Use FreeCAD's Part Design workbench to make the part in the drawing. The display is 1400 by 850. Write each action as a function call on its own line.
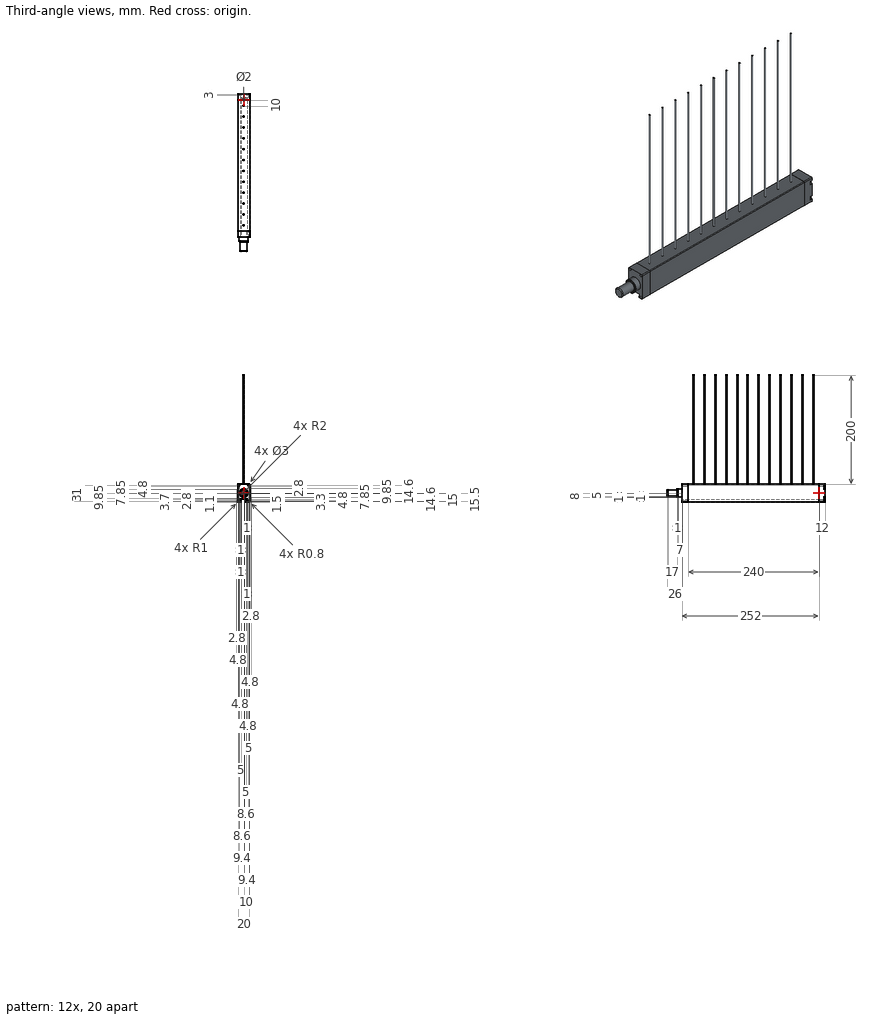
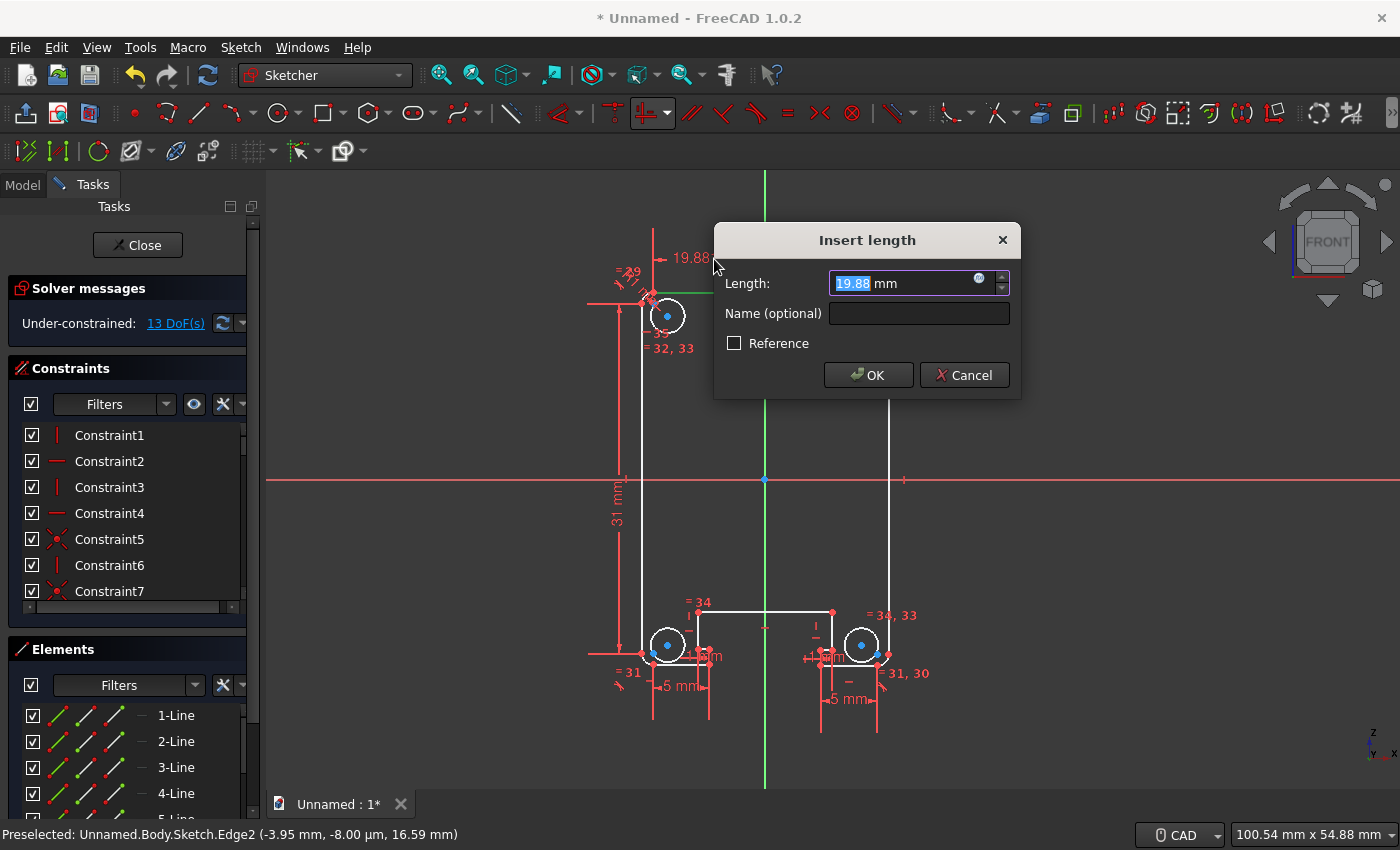
text(20)
key(Return)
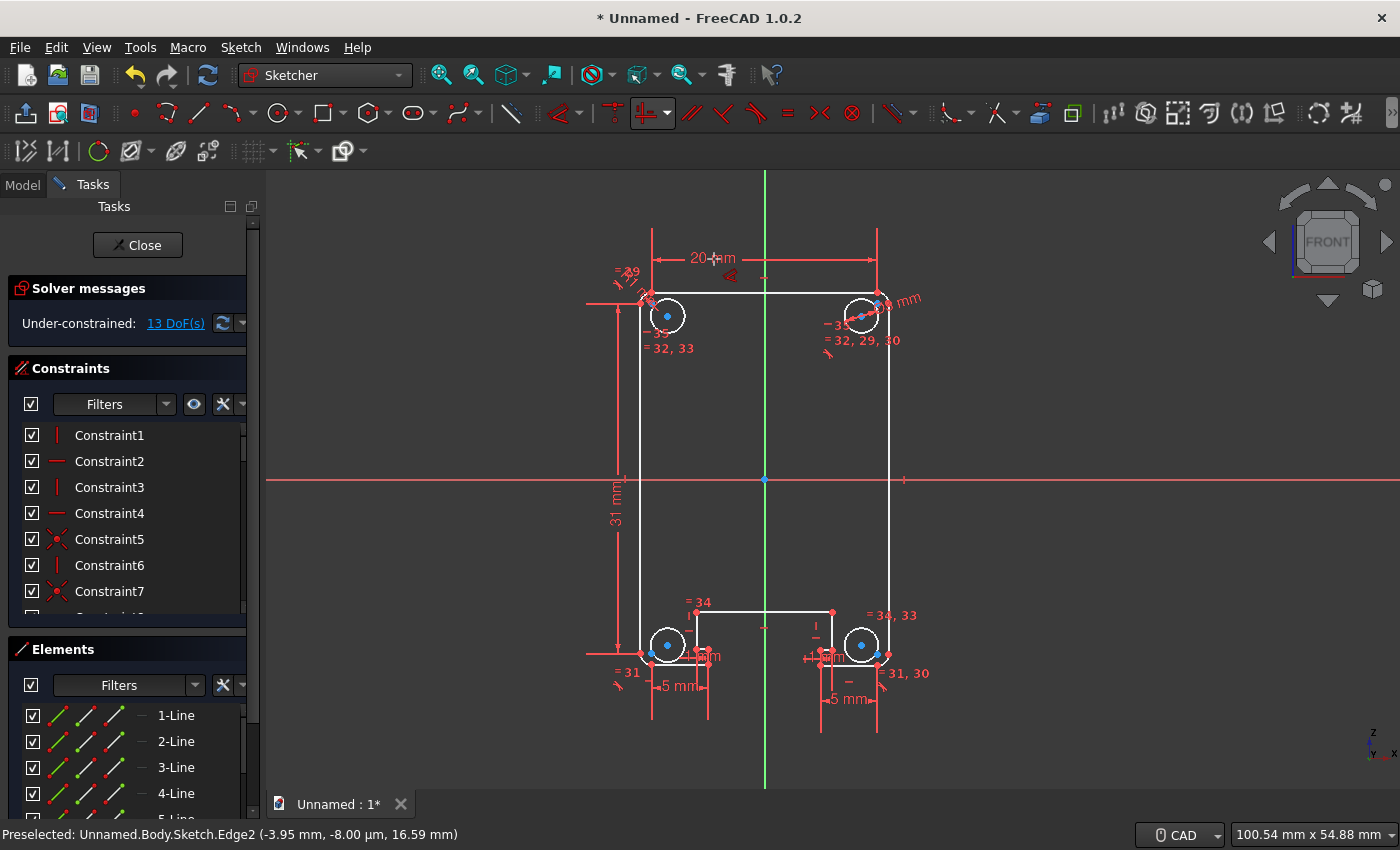
click(889, 409)
click(923, 399)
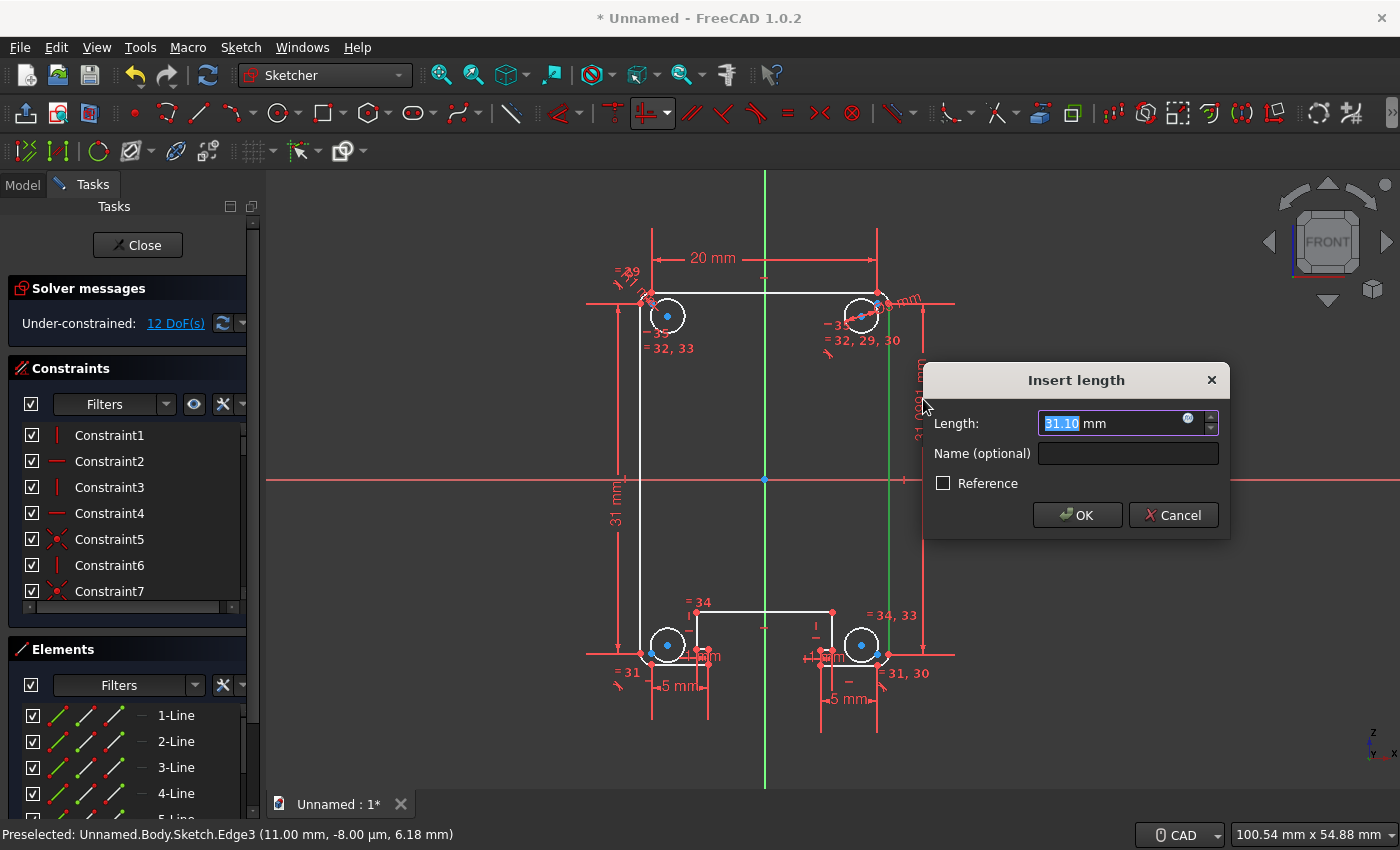
text(31)
key(Return)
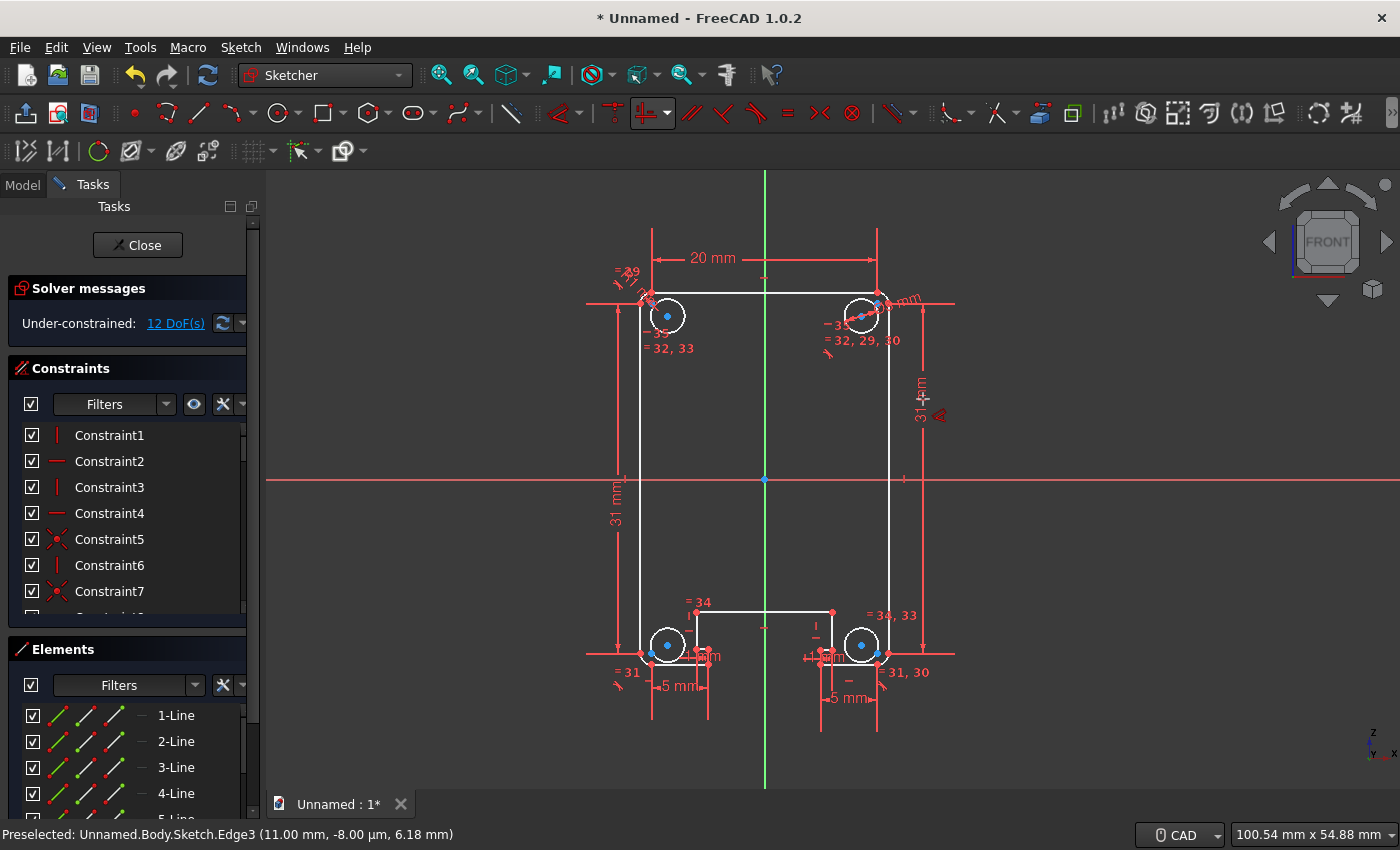
click(821, 665)
click(793, 446)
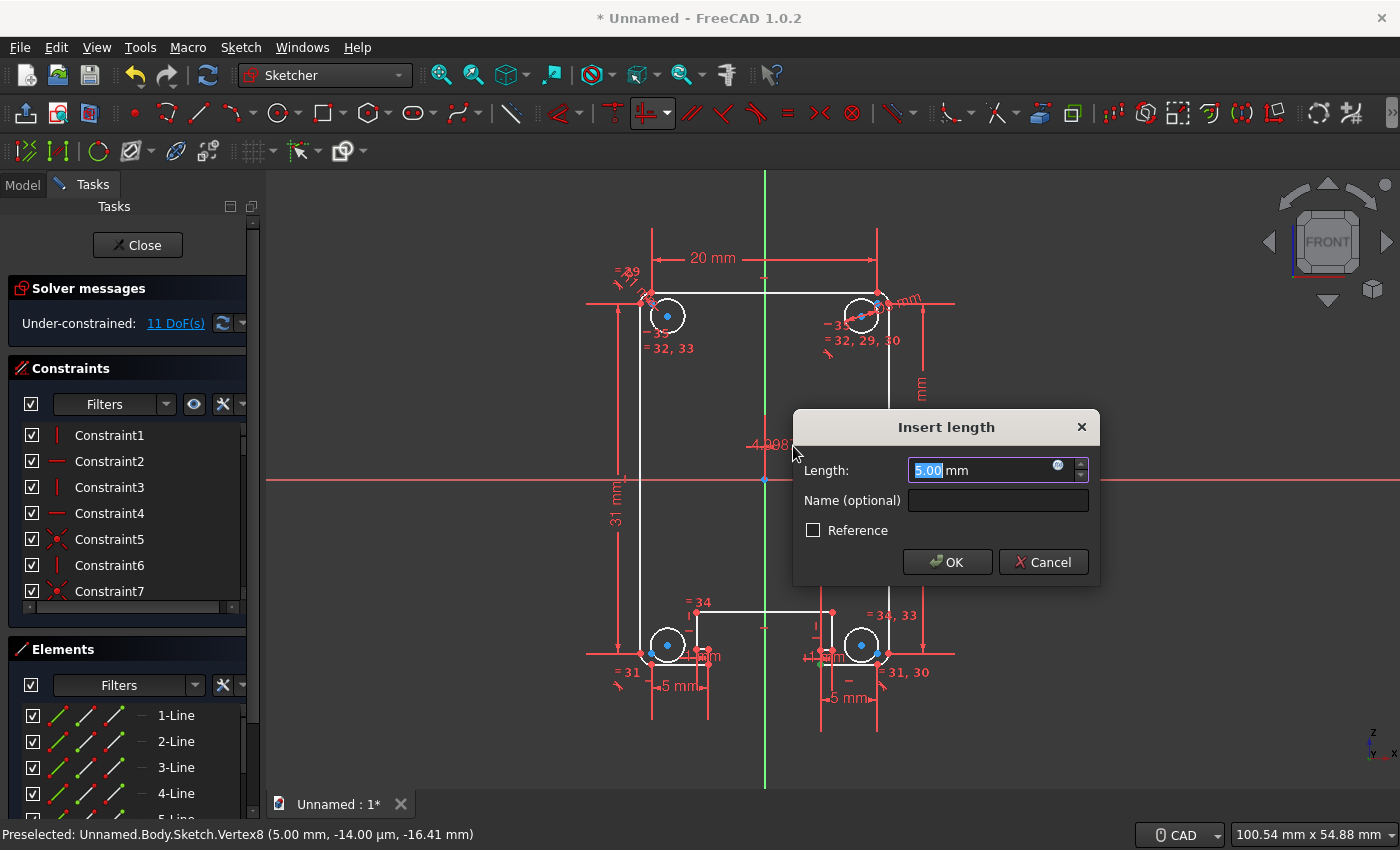
text(5)
key(Return)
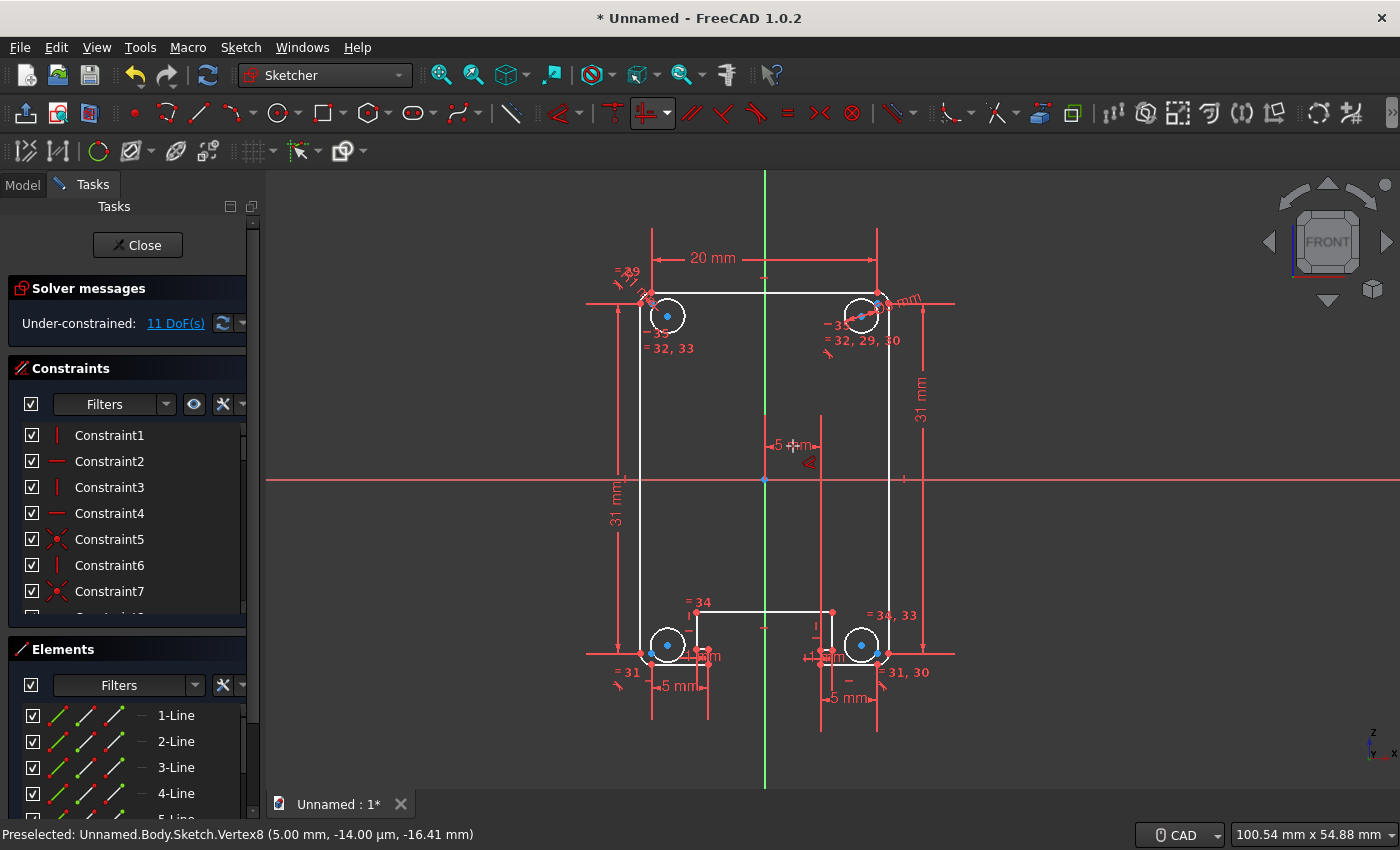
scroll(821, 657, up, 5)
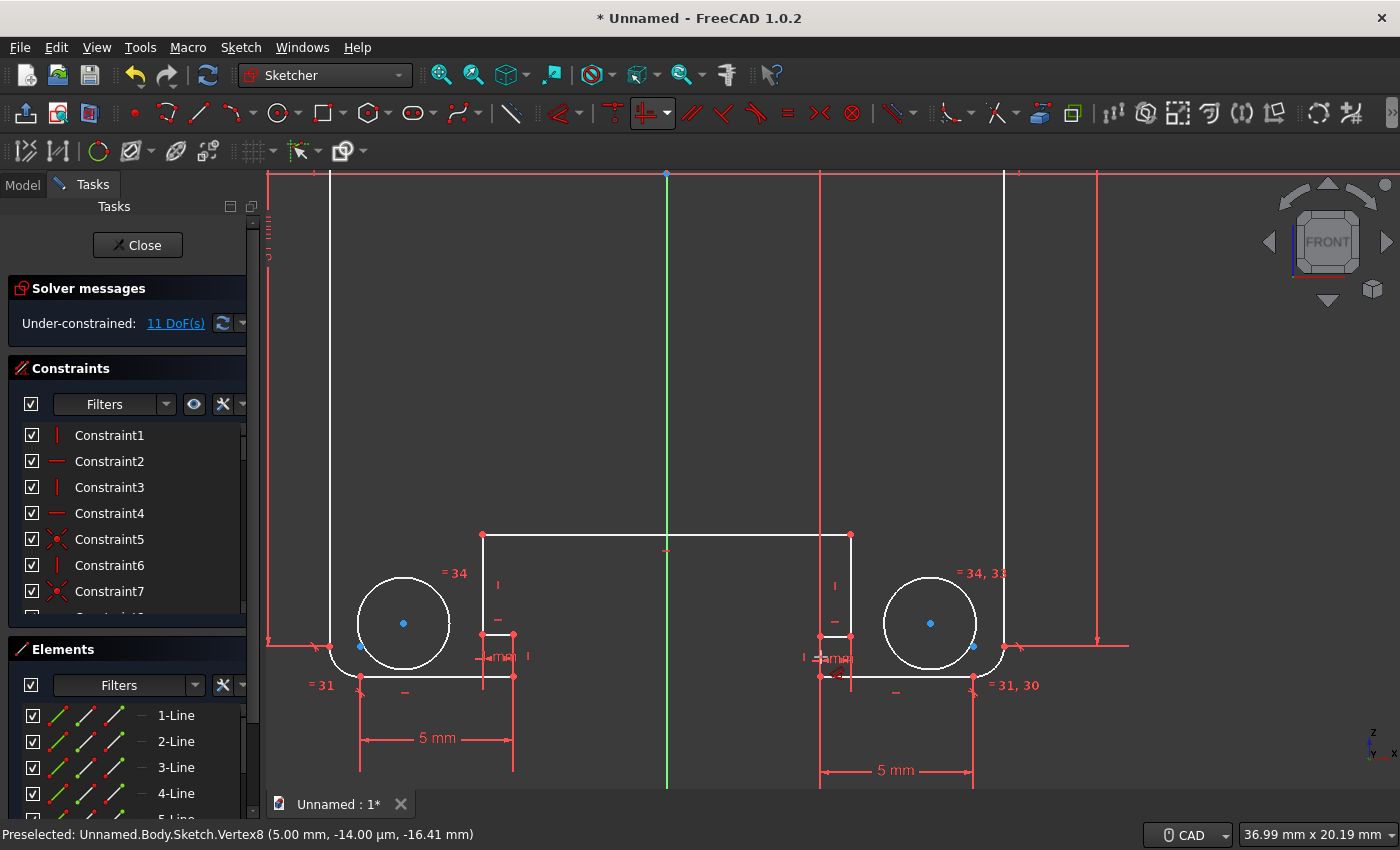
click(820, 657)
click(762, 657)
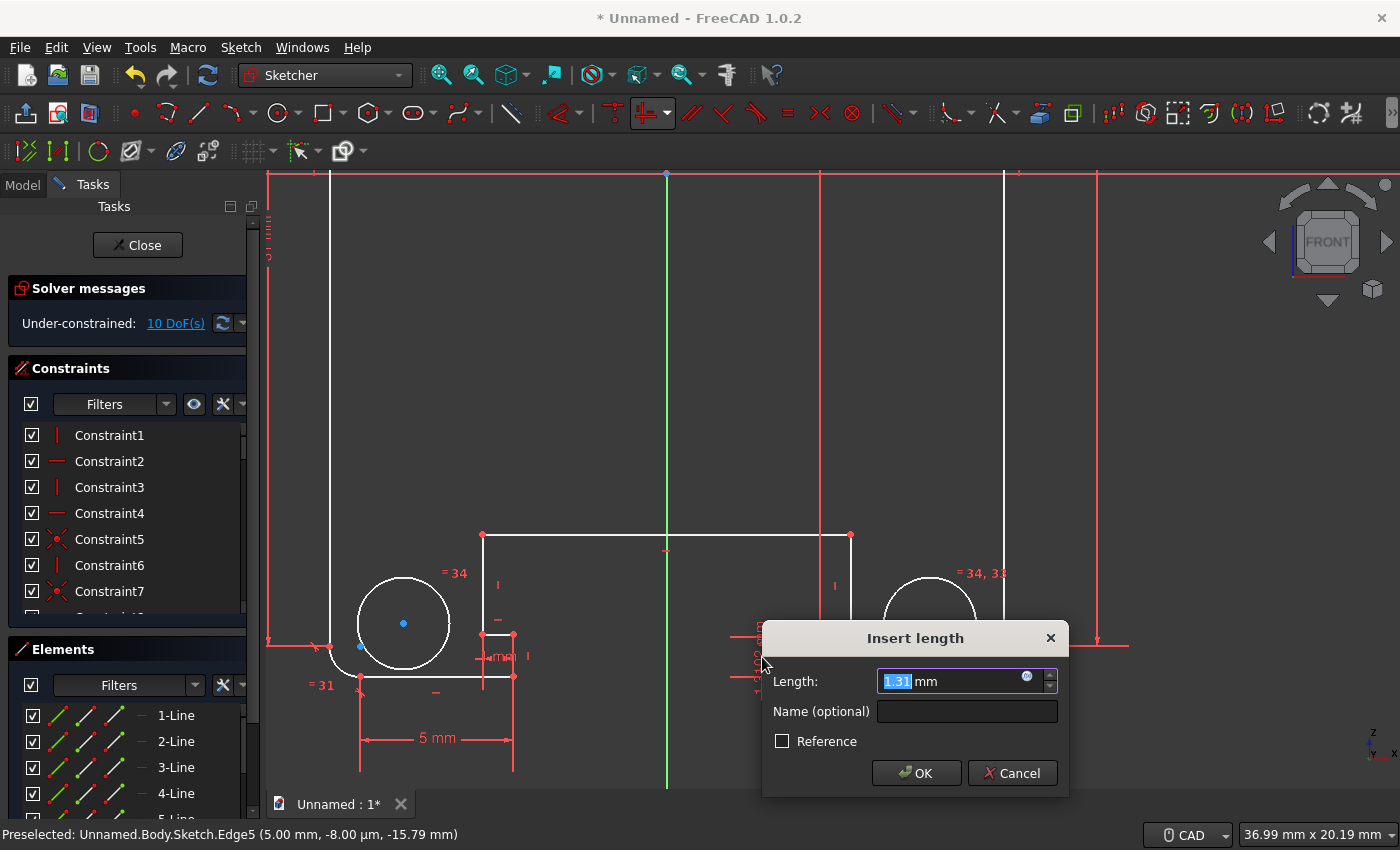
text(1.5)
key(Return)